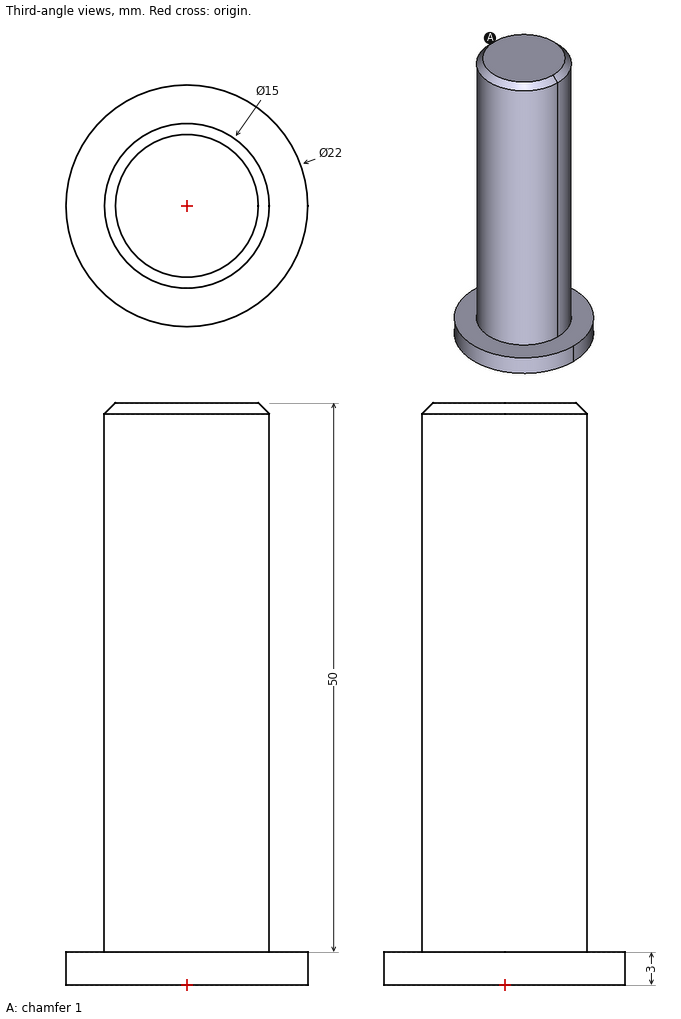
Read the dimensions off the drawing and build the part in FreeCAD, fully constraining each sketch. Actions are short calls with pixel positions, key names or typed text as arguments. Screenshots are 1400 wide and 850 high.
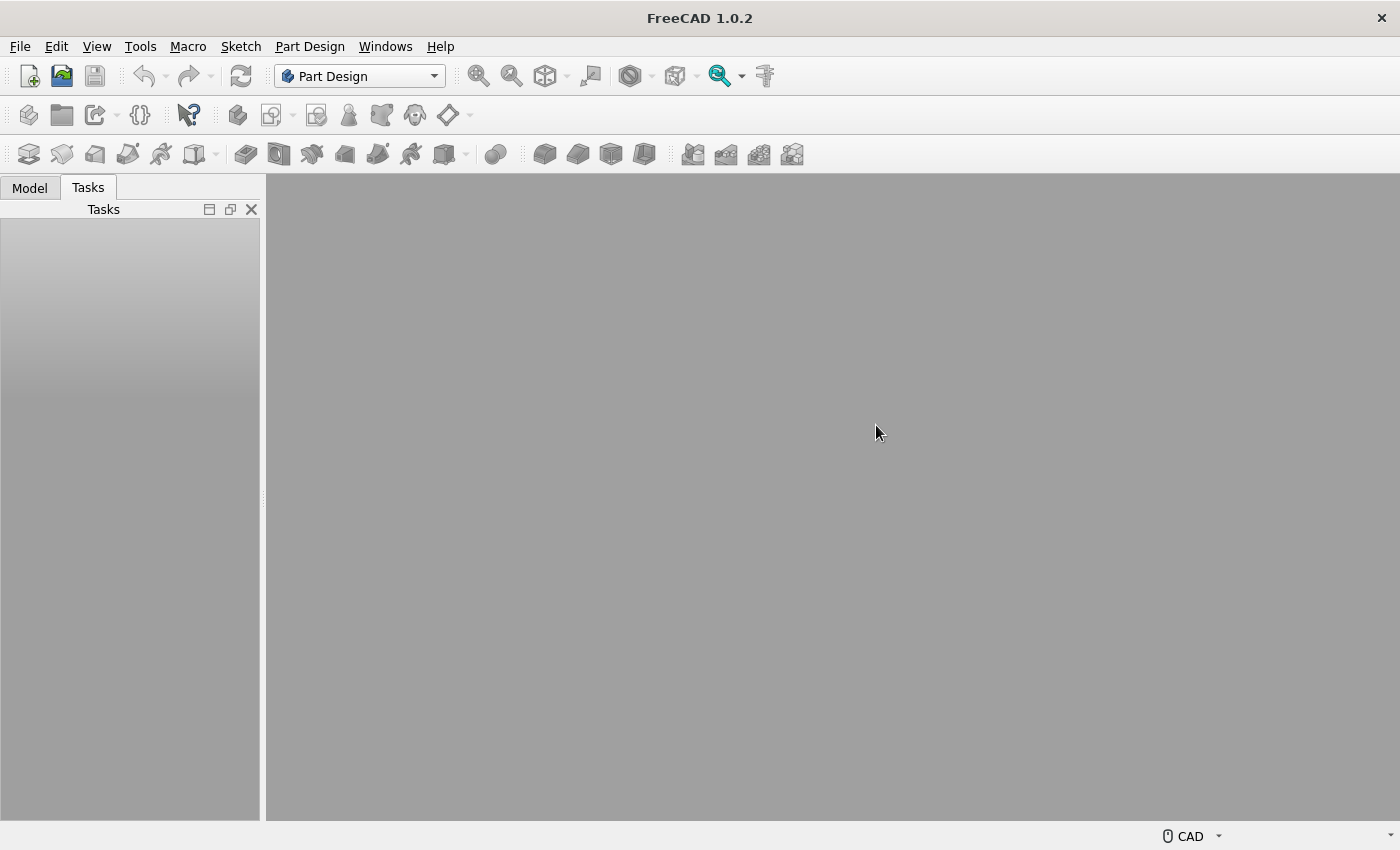
click(29, 76)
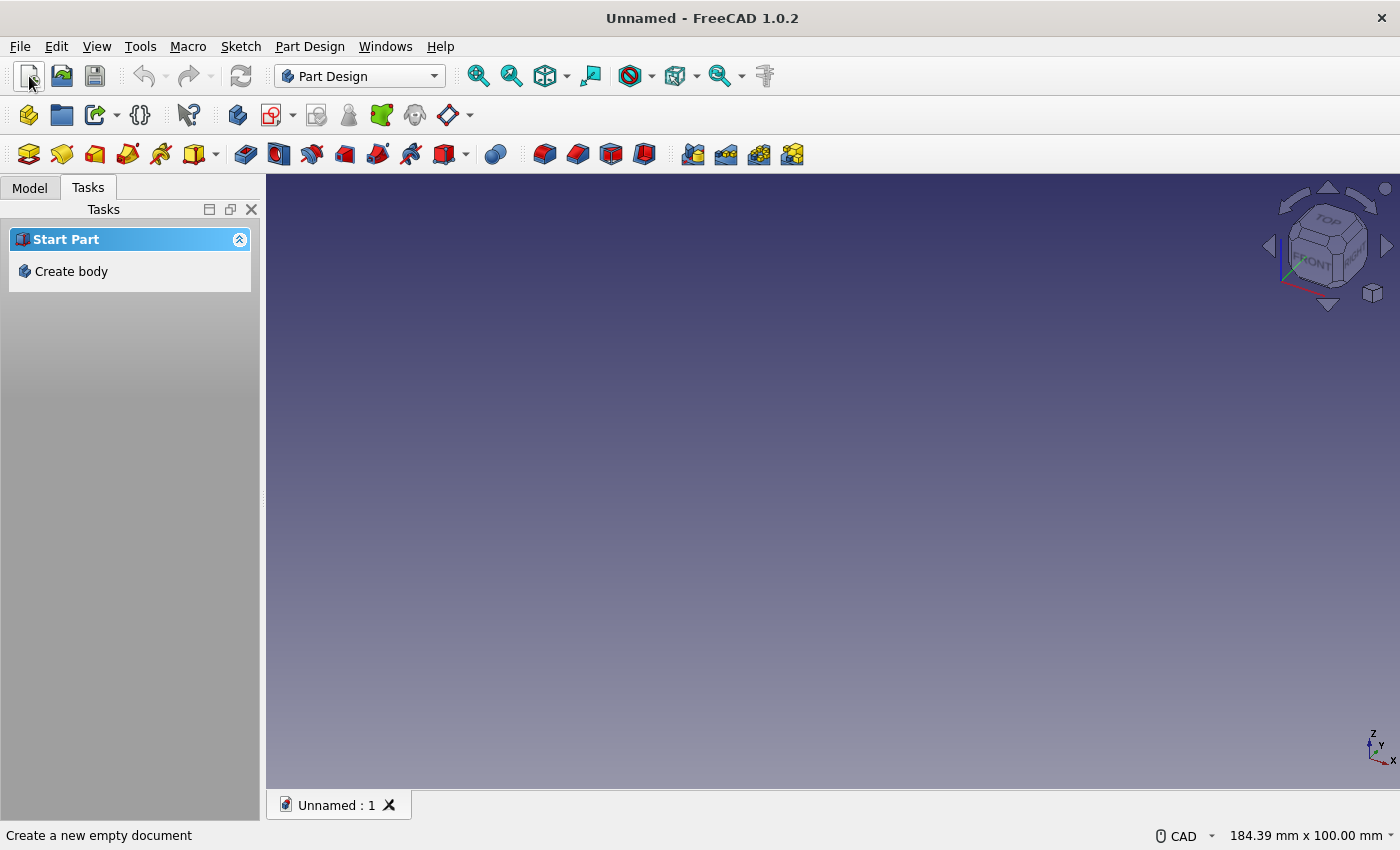
click(270, 116)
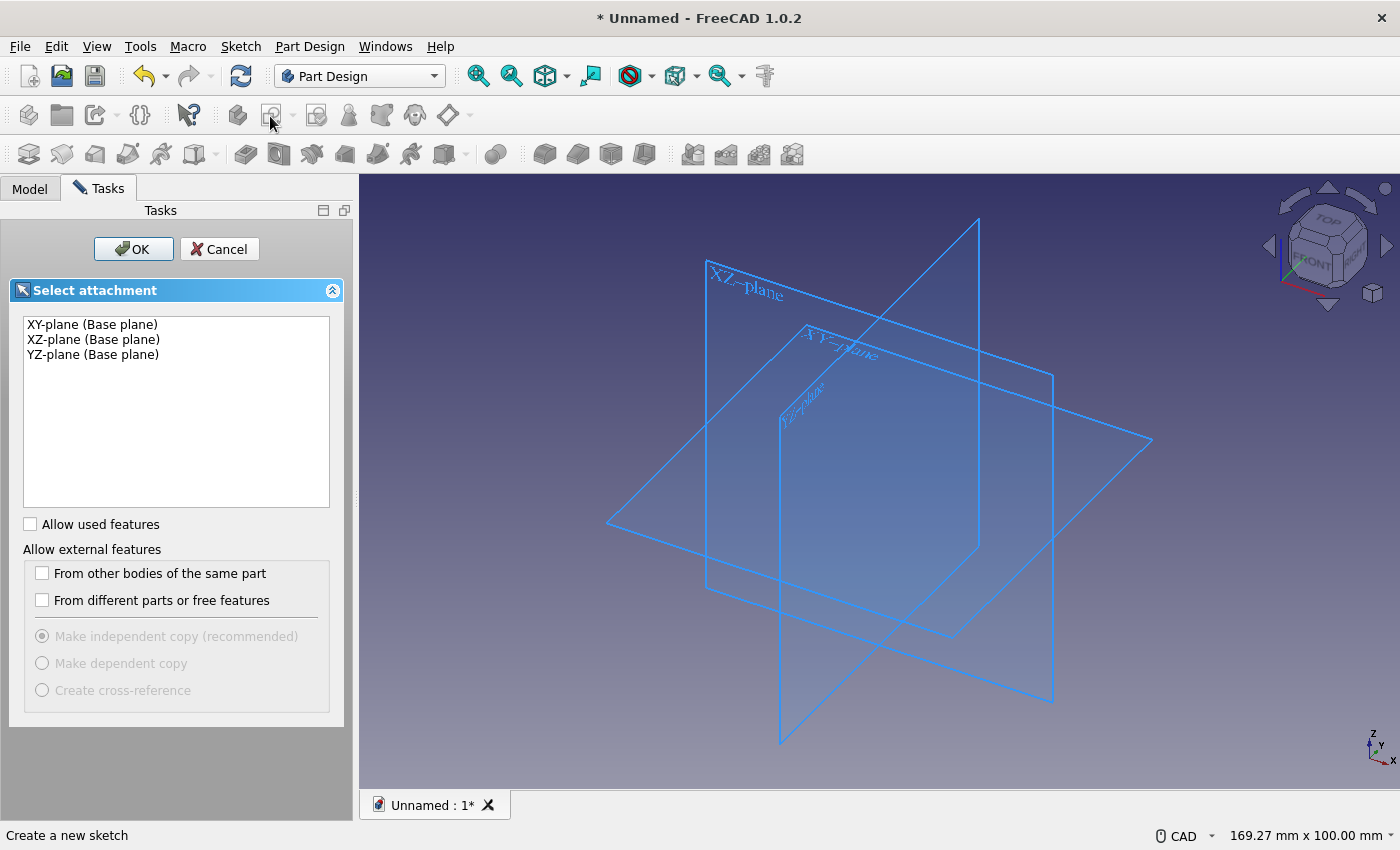
click(84, 324)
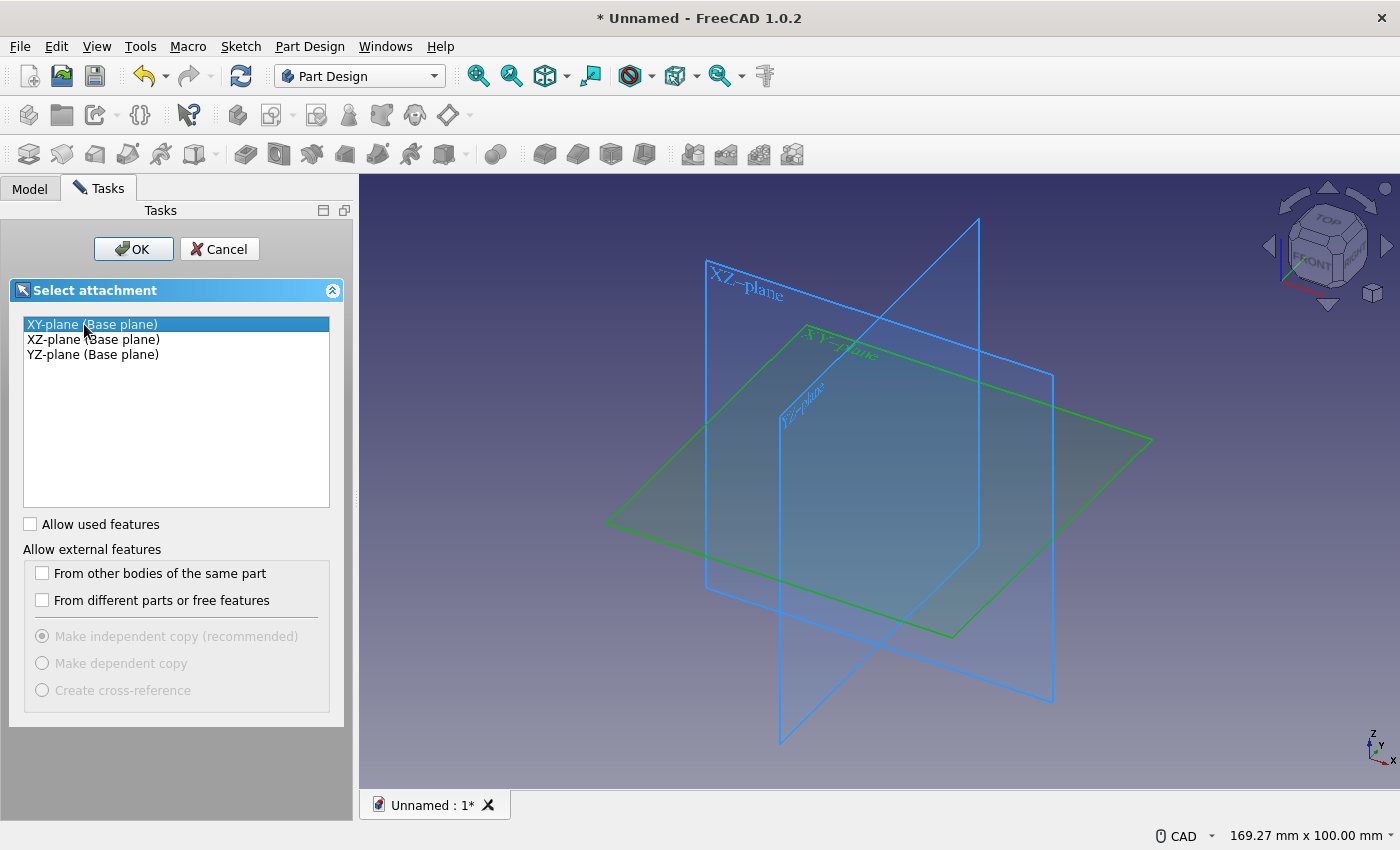
click(134, 249)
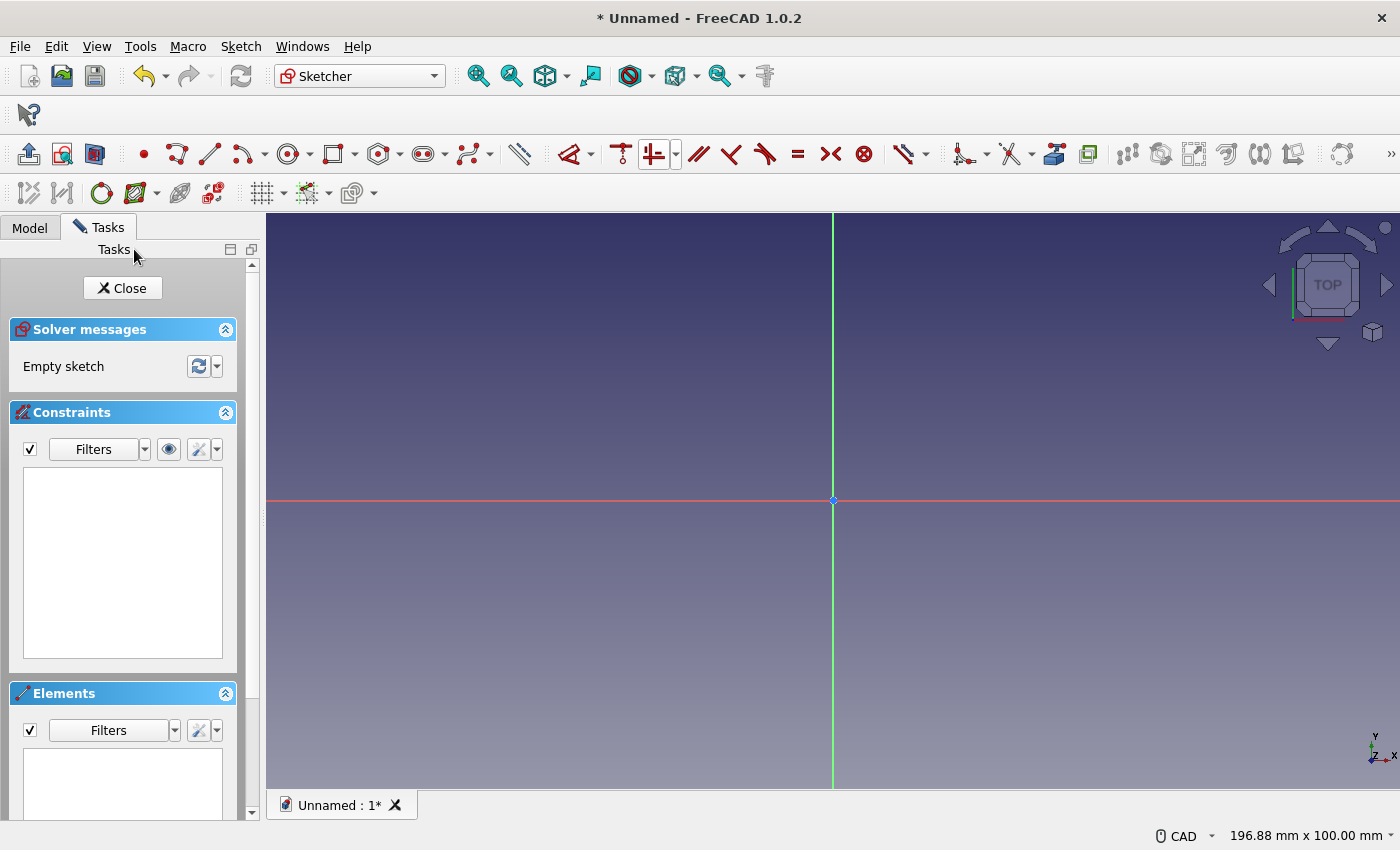
scroll(873, 501, up, 5)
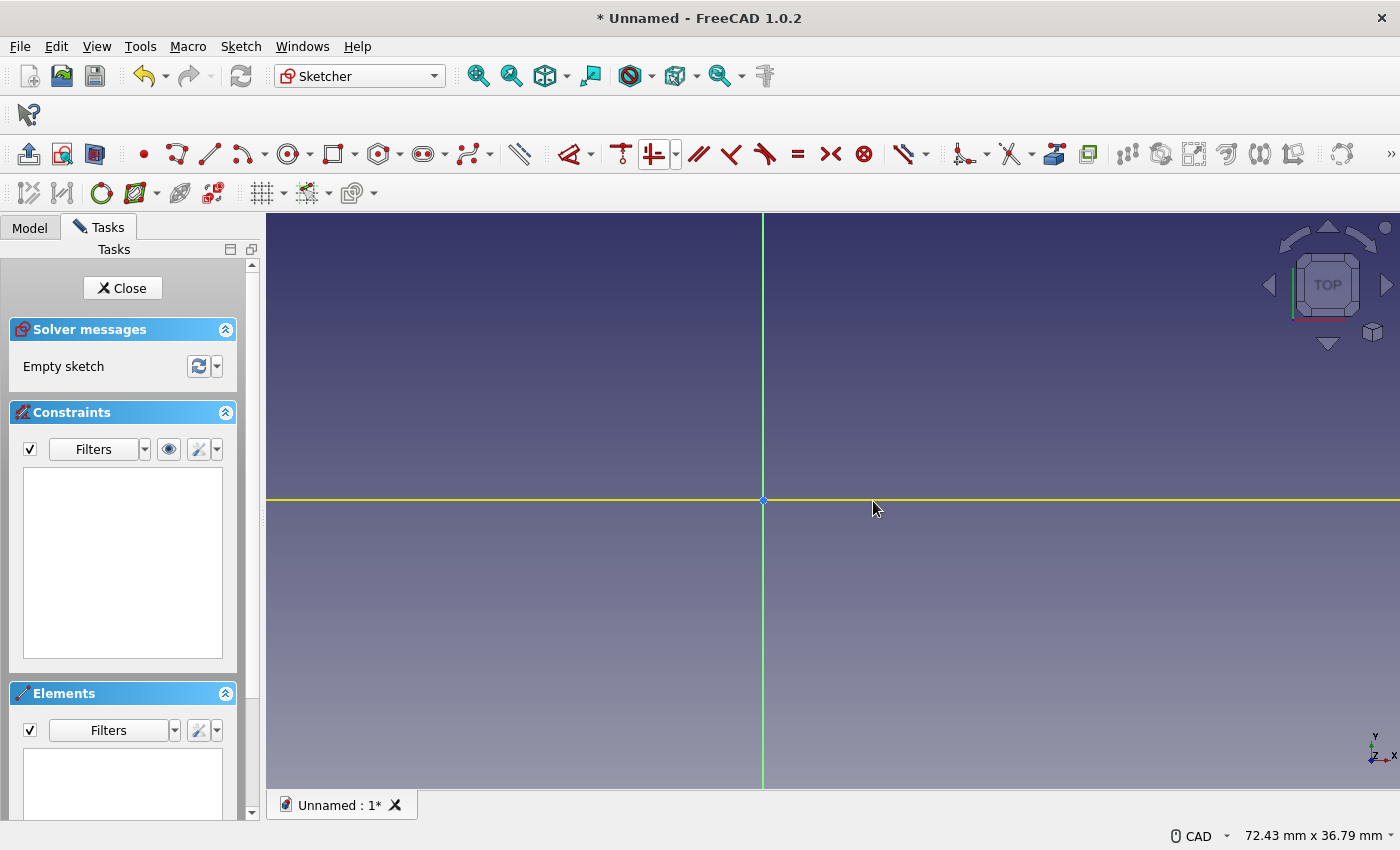
click(288, 154)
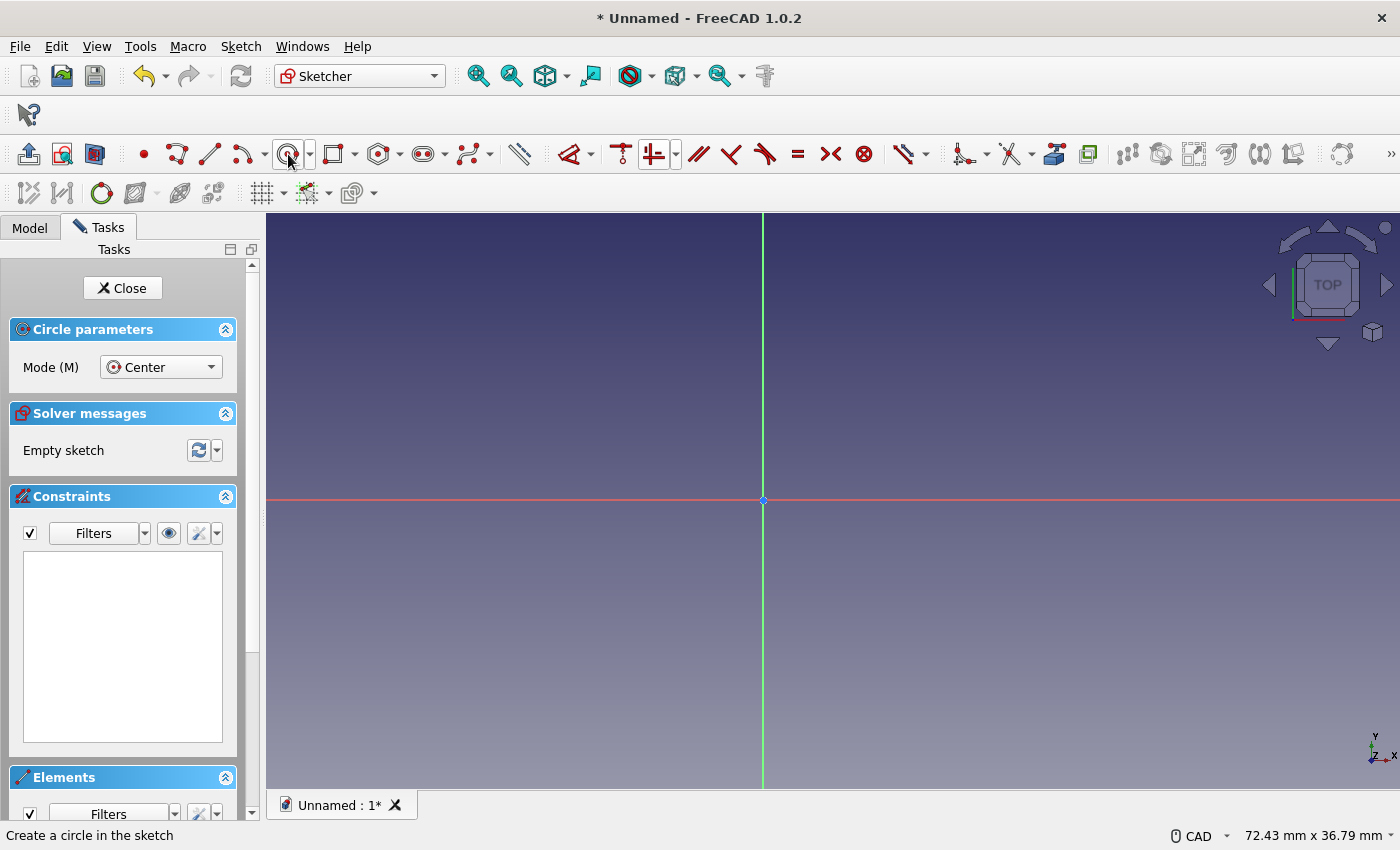
click(763, 500)
move(885, 378)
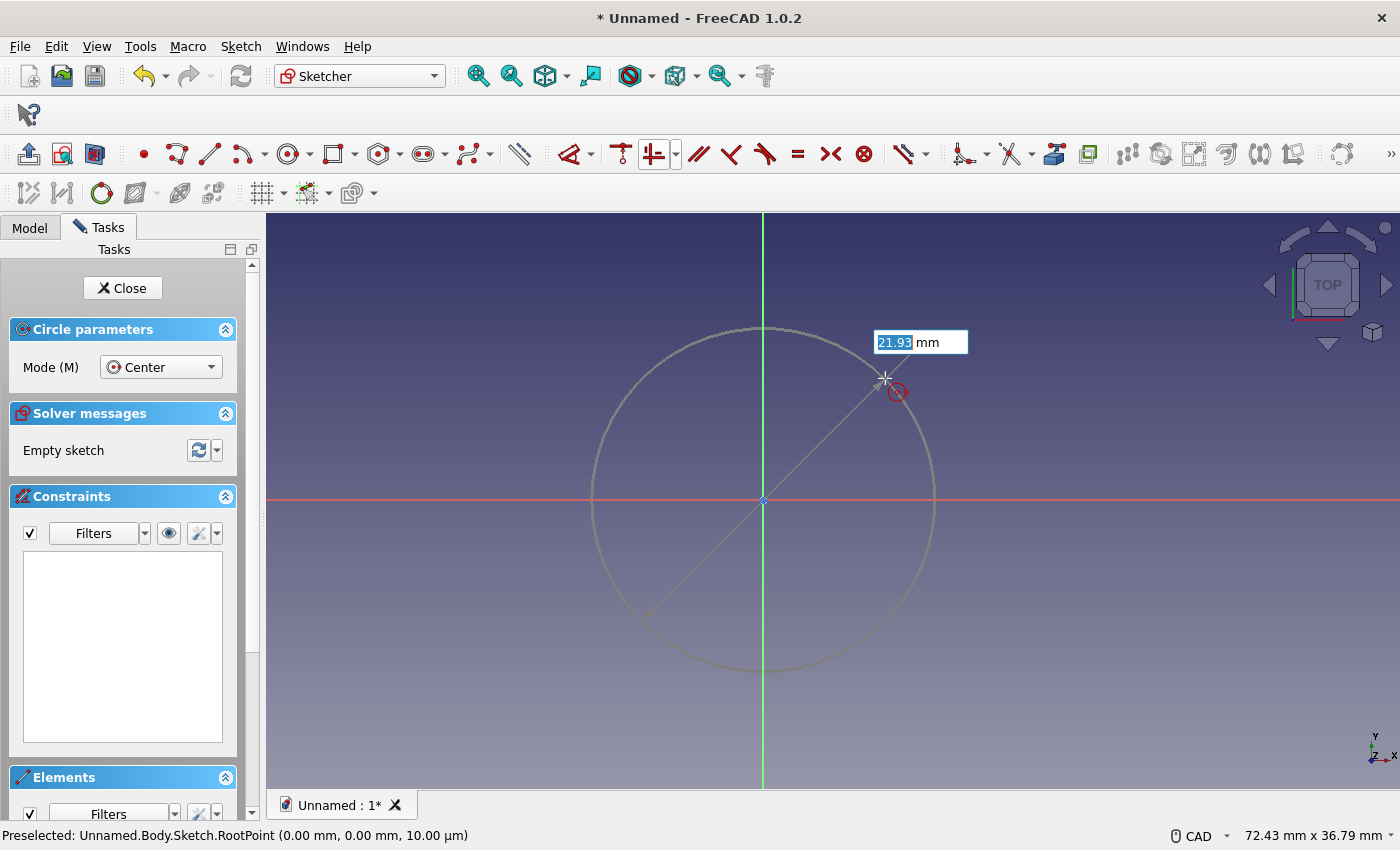
text(22)
key(Return)
key(Escape)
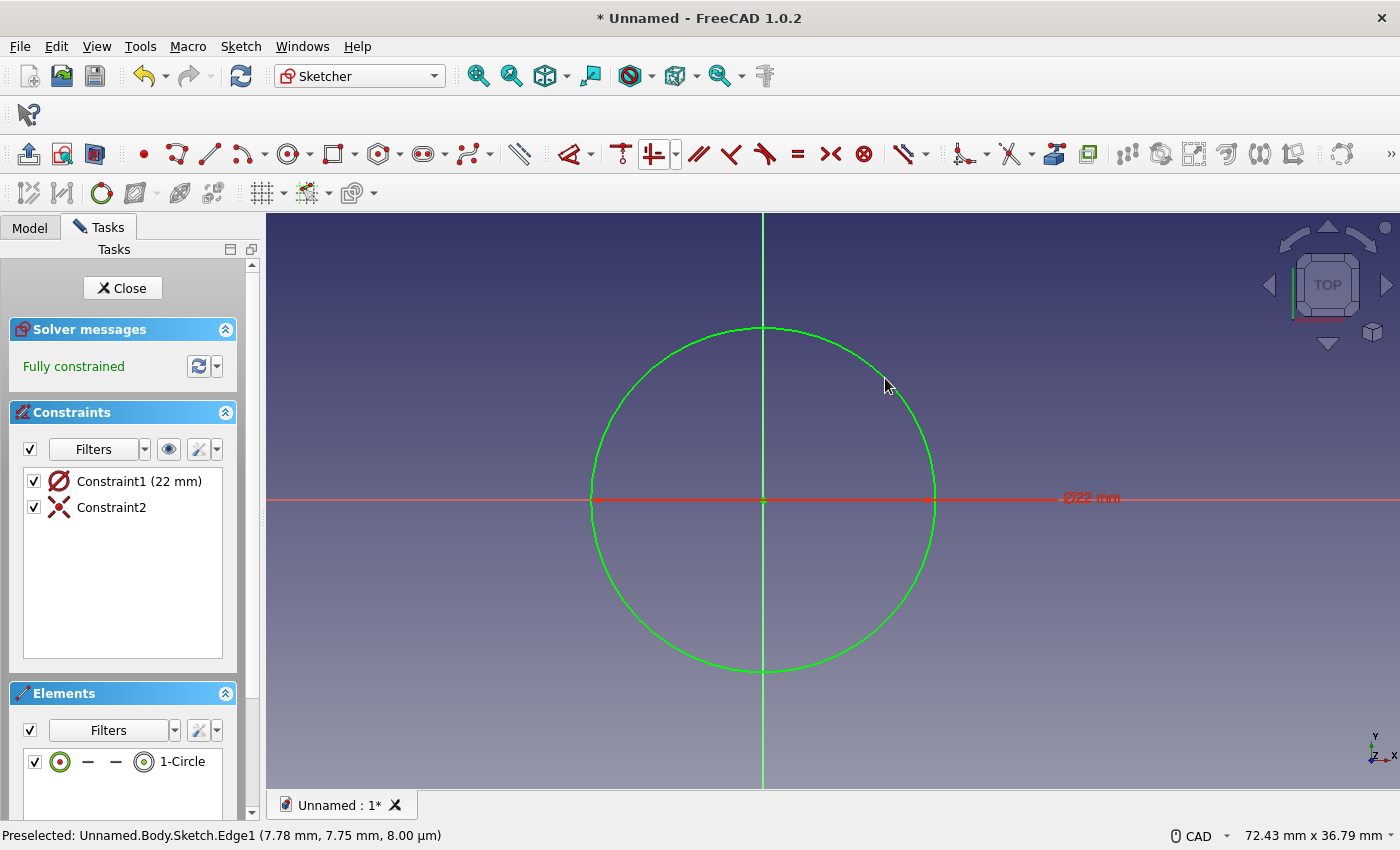
click(123, 288)